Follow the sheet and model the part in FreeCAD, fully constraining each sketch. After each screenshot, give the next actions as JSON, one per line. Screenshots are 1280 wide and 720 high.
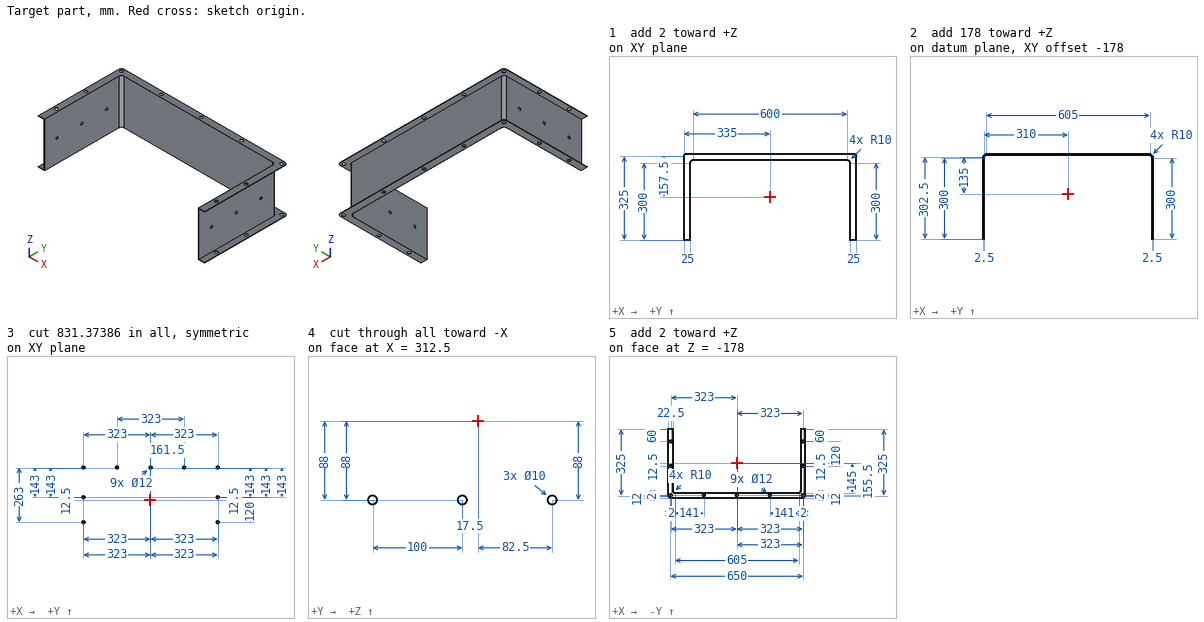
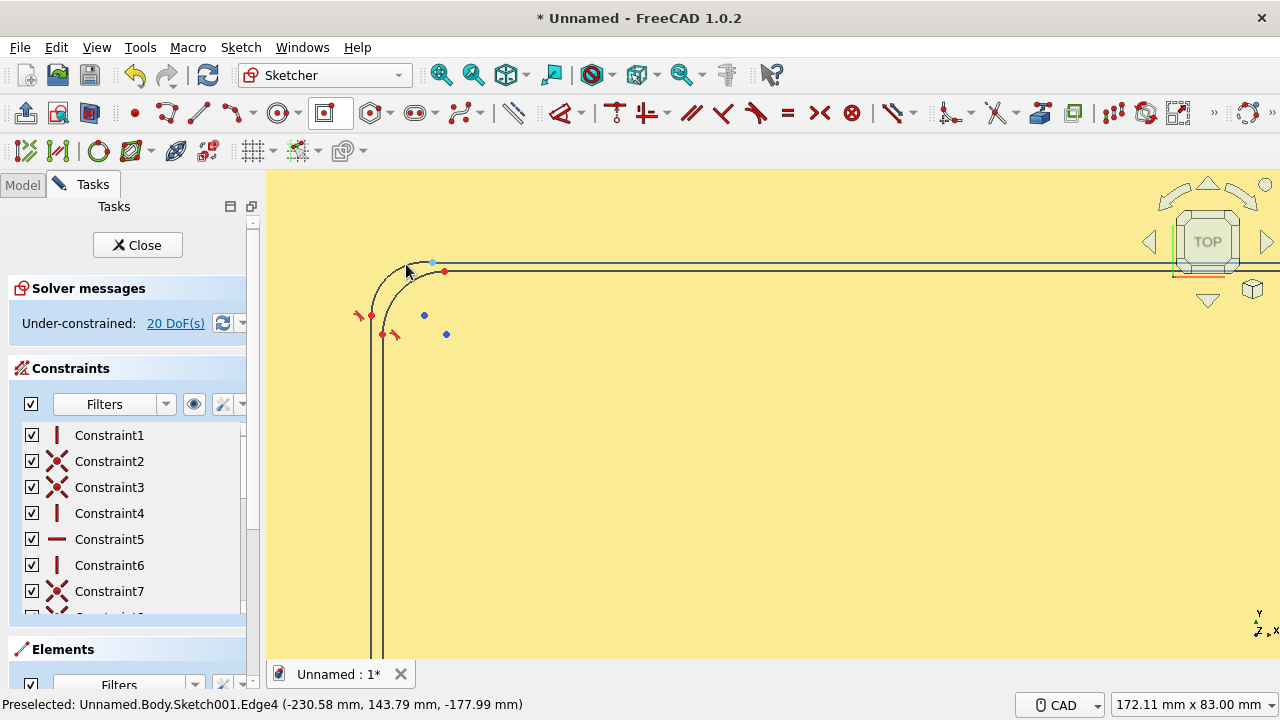
{"action": "left_click", "coordinate": [405, 266]}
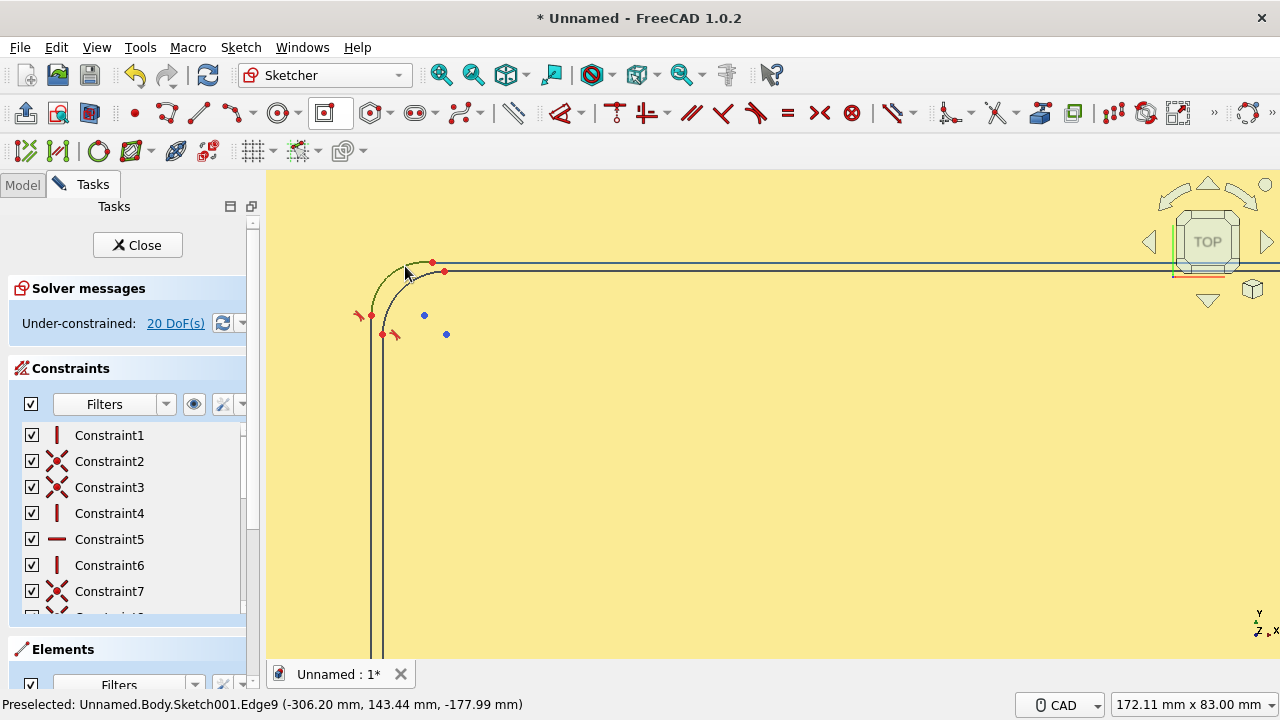
{"action": "left_click", "coordinate": [756, 114]}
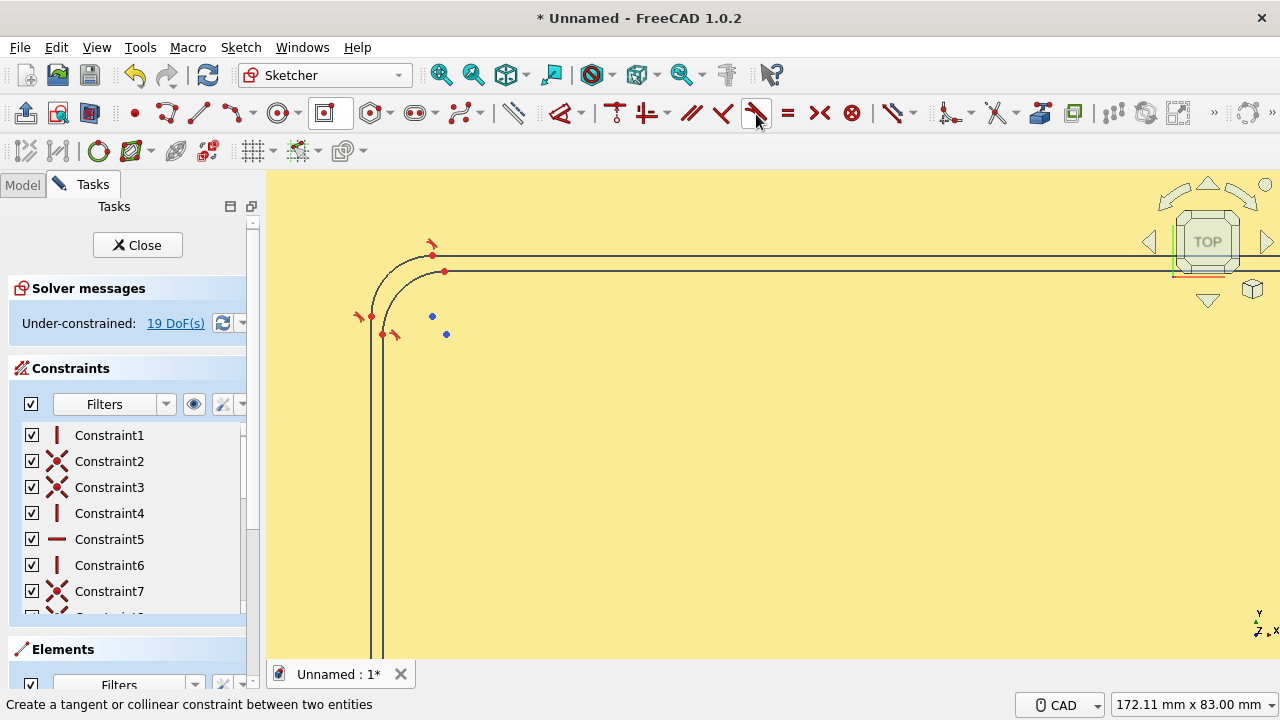
{"action": "scroll", "coordinate": [406, 264], "scroll_direction": "down", "scroll_amount": 9}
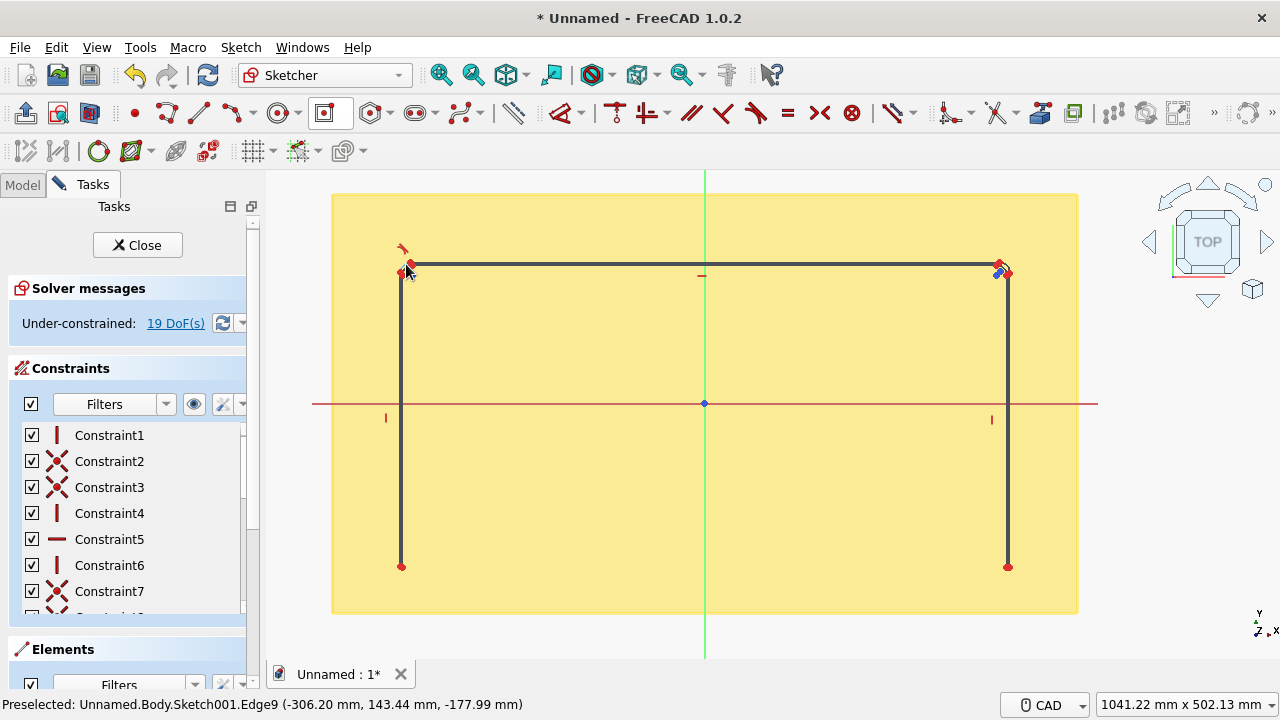
{"action": "scroll", "coordinate": [587, 263], "scroll_direction": "up", "scroll_amount": 9}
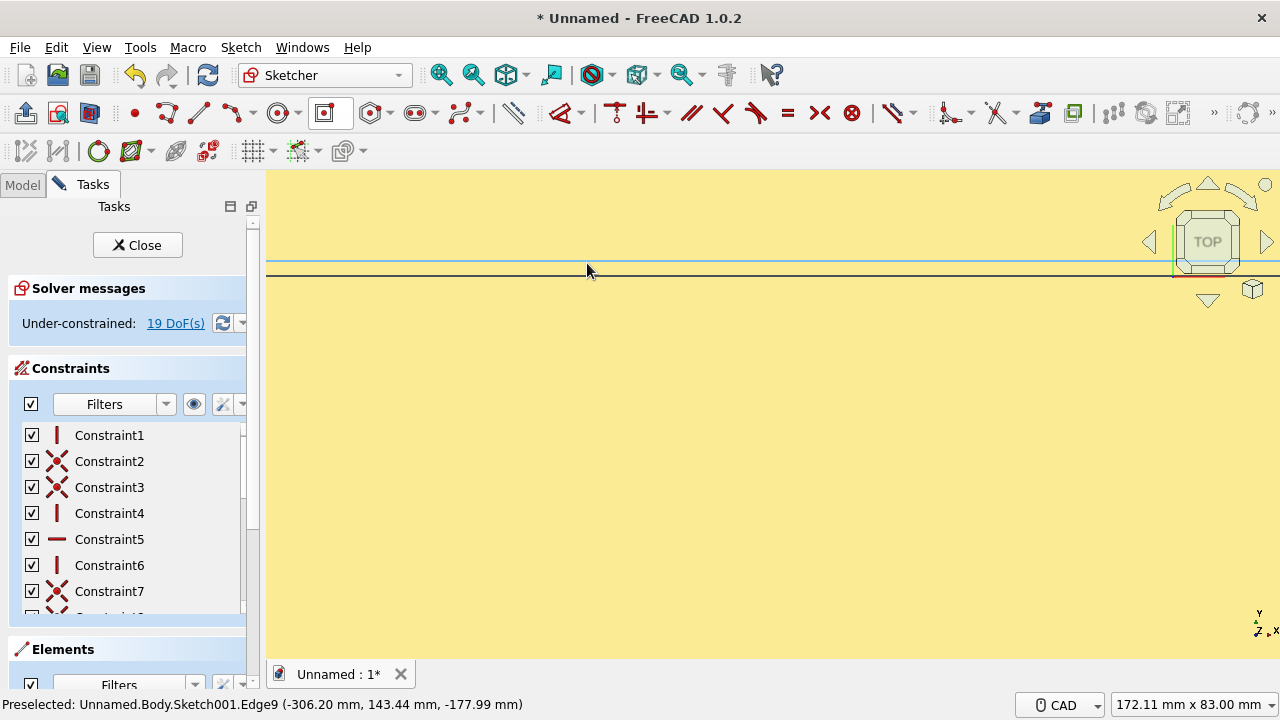
{"action": "left_click", "coordinate": [586, 261]}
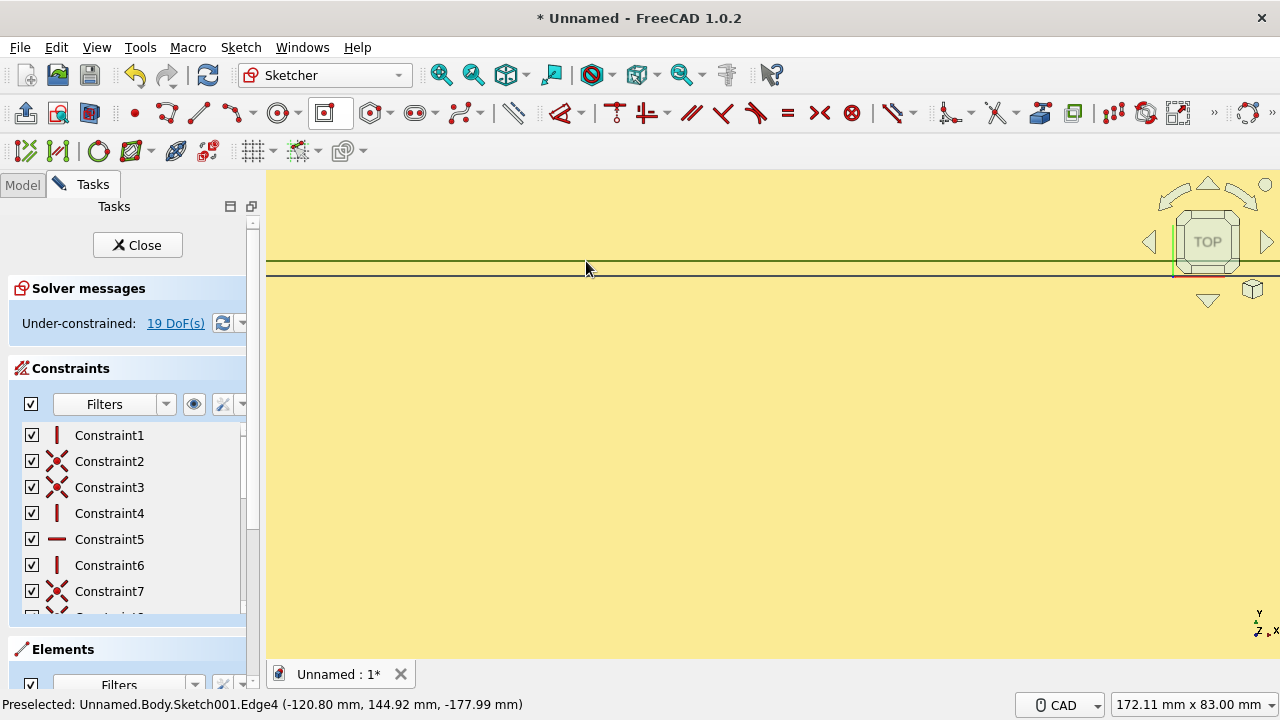
{"action": "scroll", "coordinate": [587, 263], "scroll_direction": "down", "scroll_amount": 9}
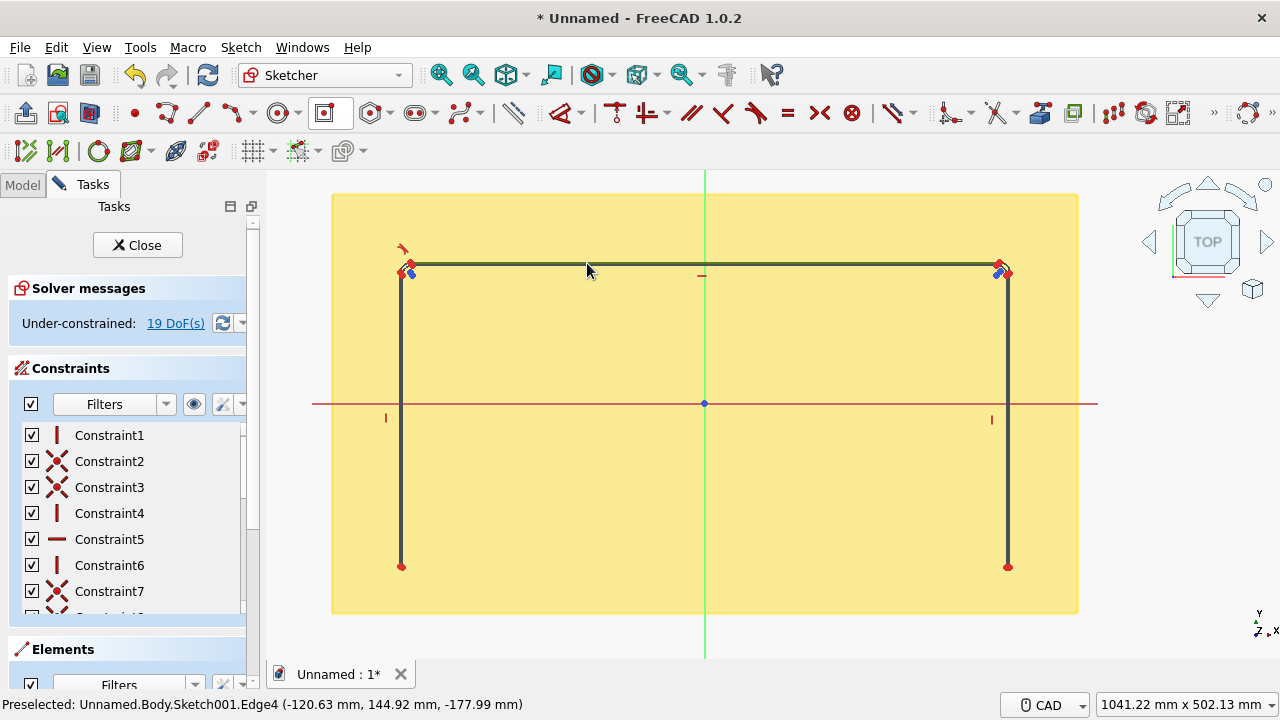
{"action": "scroll", "coordinate": [1009, 269], "scroll_direction": "up", "scroll_amount": 7}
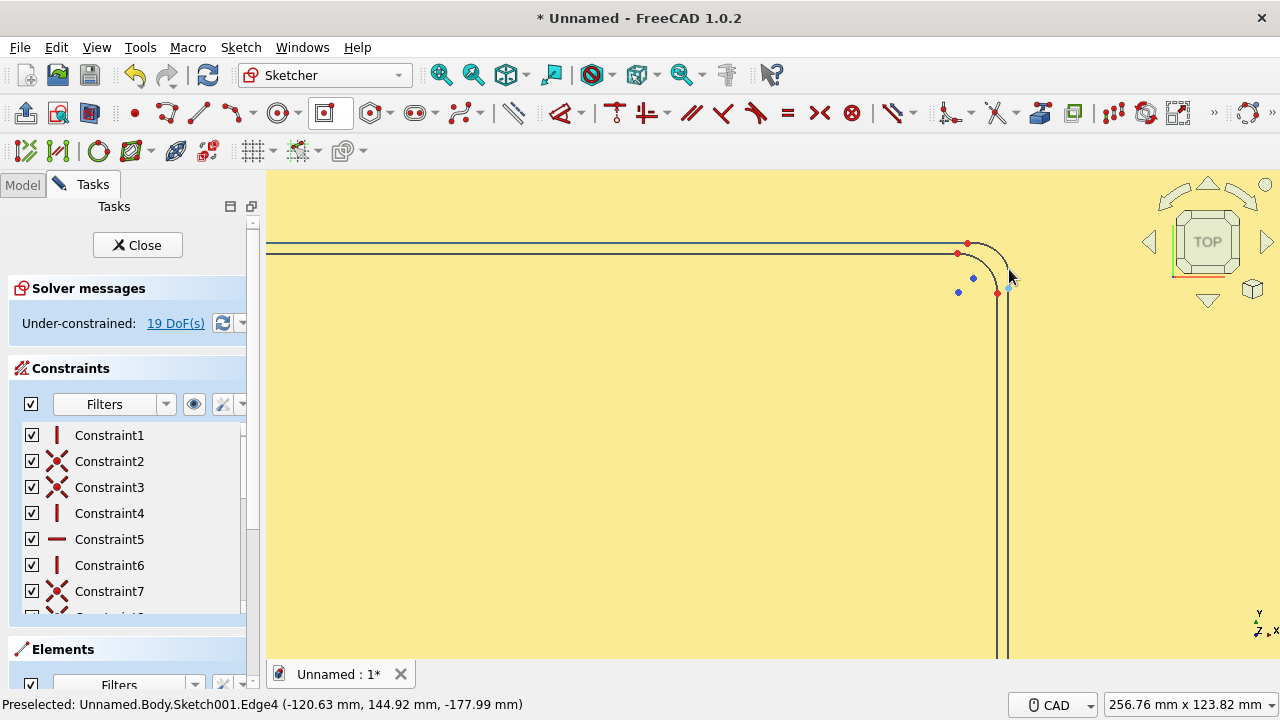
{"action": "left_click", "coordinate": [1008, 267]}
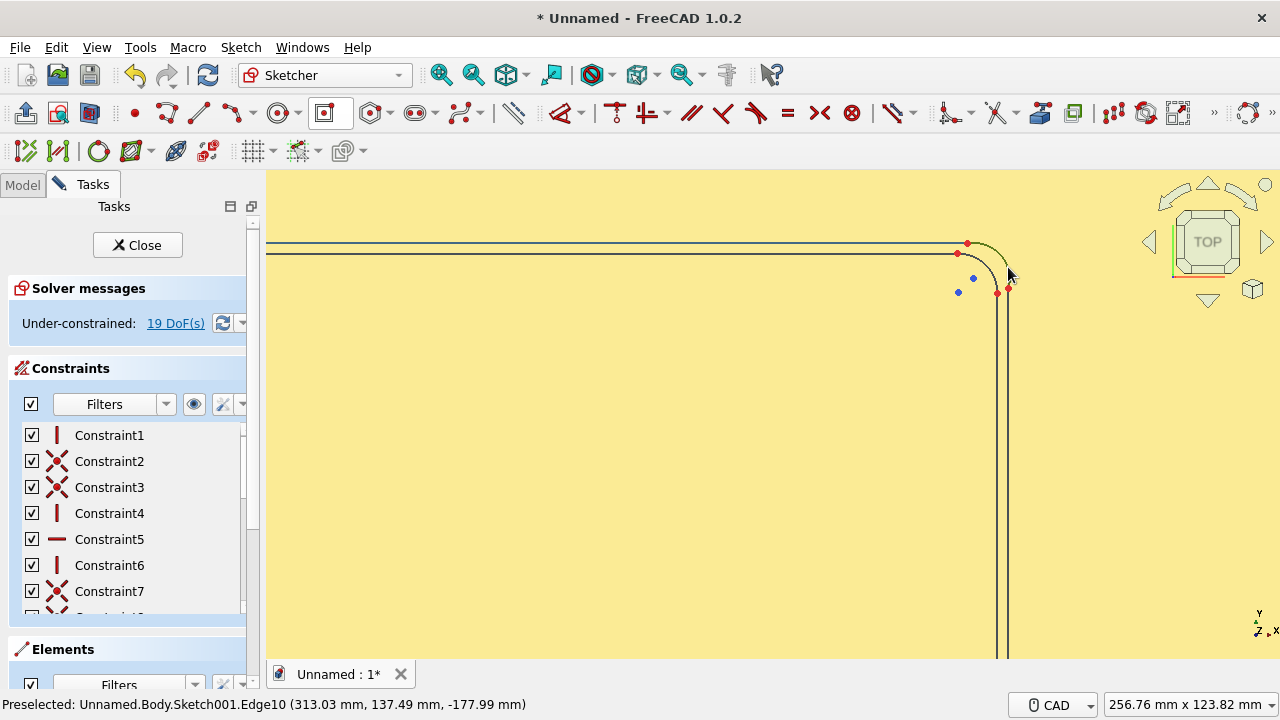
{"action": "left_click", "coordinate": [756, 114]}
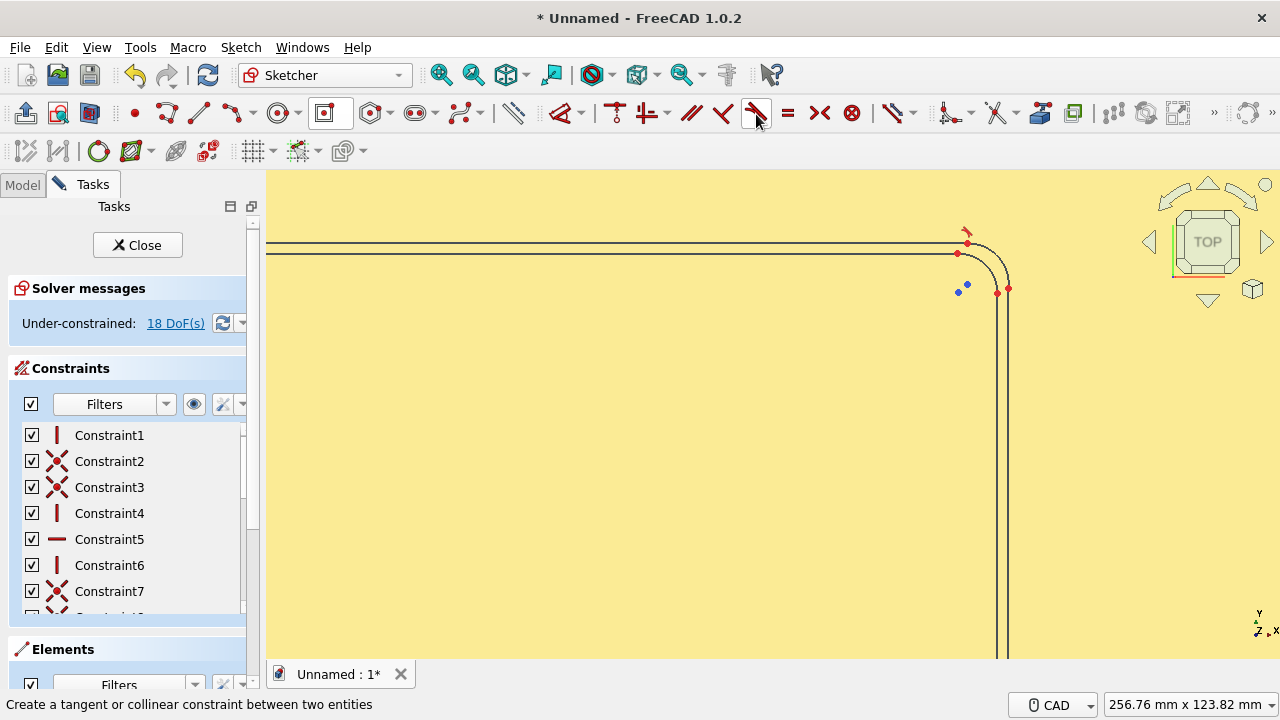
{"action": "scroll", "coordinate": [1008, 527], "scroll_direction": "up", "scroll_amount": 2}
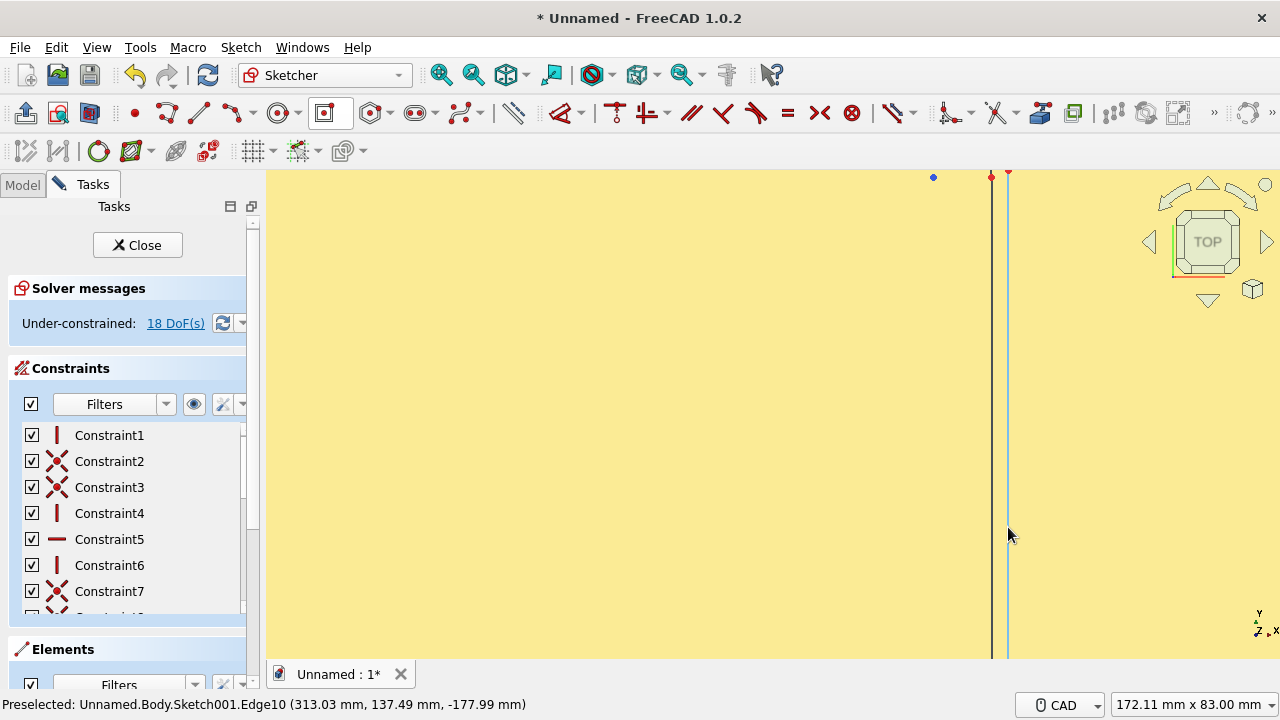
{"action": "left_click", "coordinate": [1008, 526]}